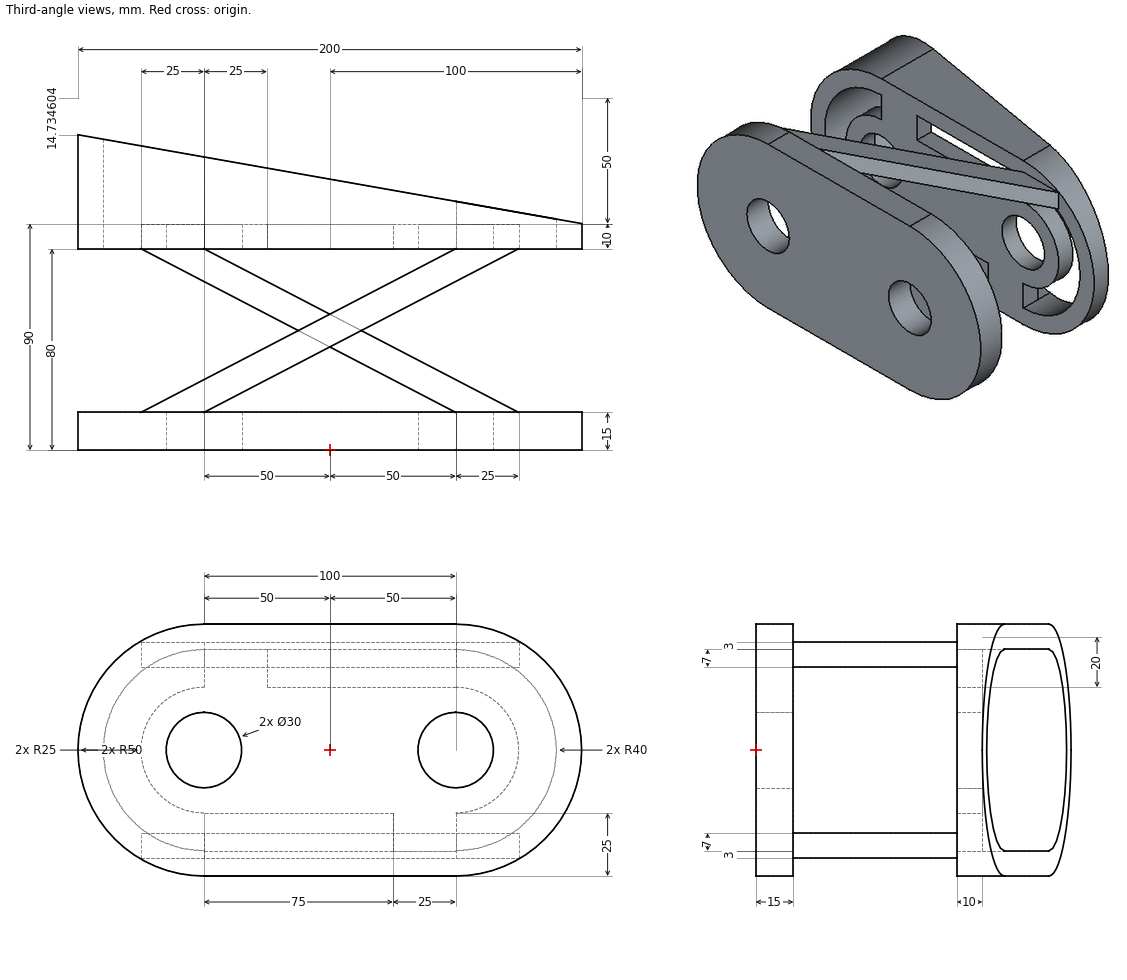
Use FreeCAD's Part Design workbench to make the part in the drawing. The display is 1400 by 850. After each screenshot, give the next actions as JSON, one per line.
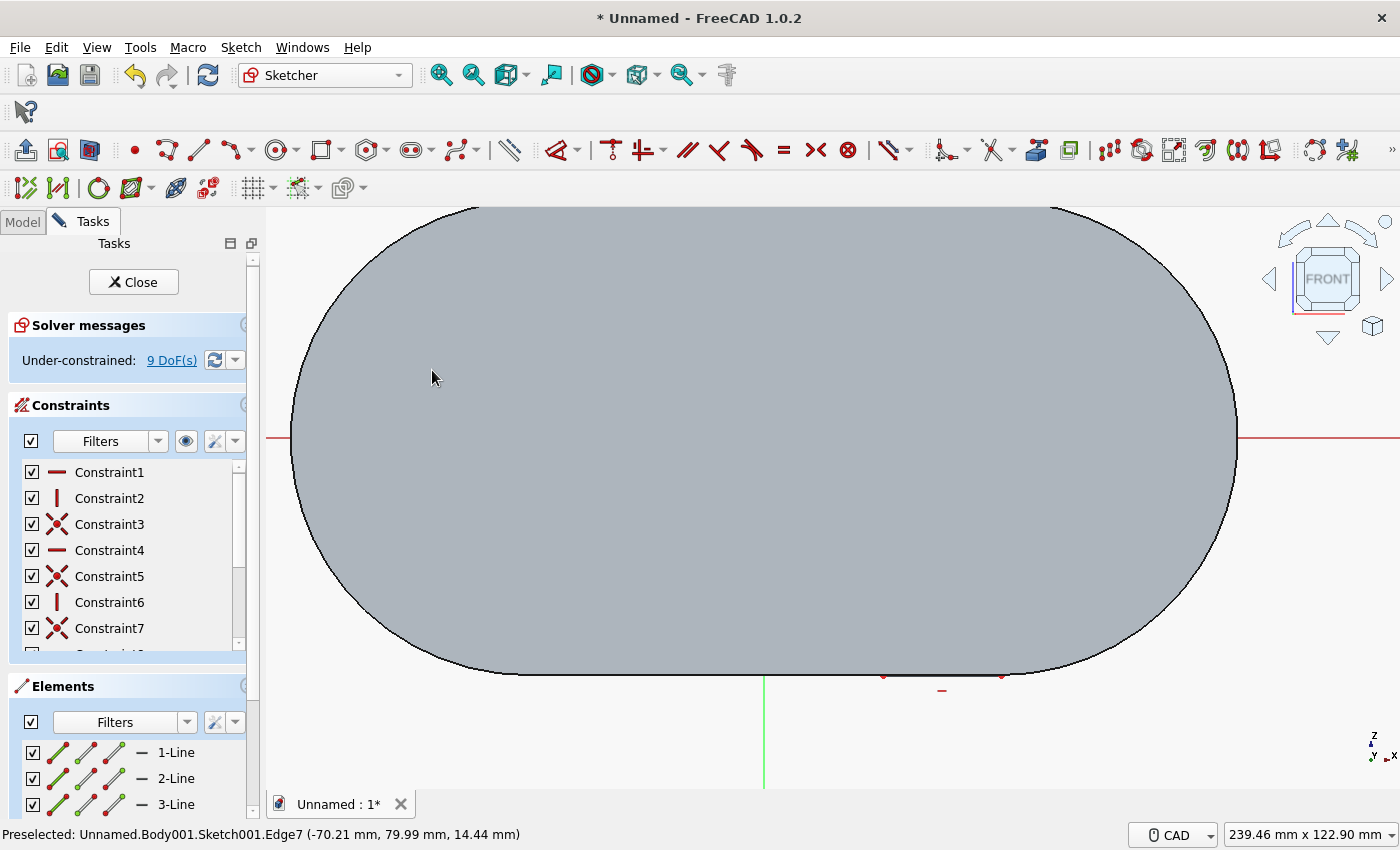
{"action": "left_click", "coordinate": [752, 150]}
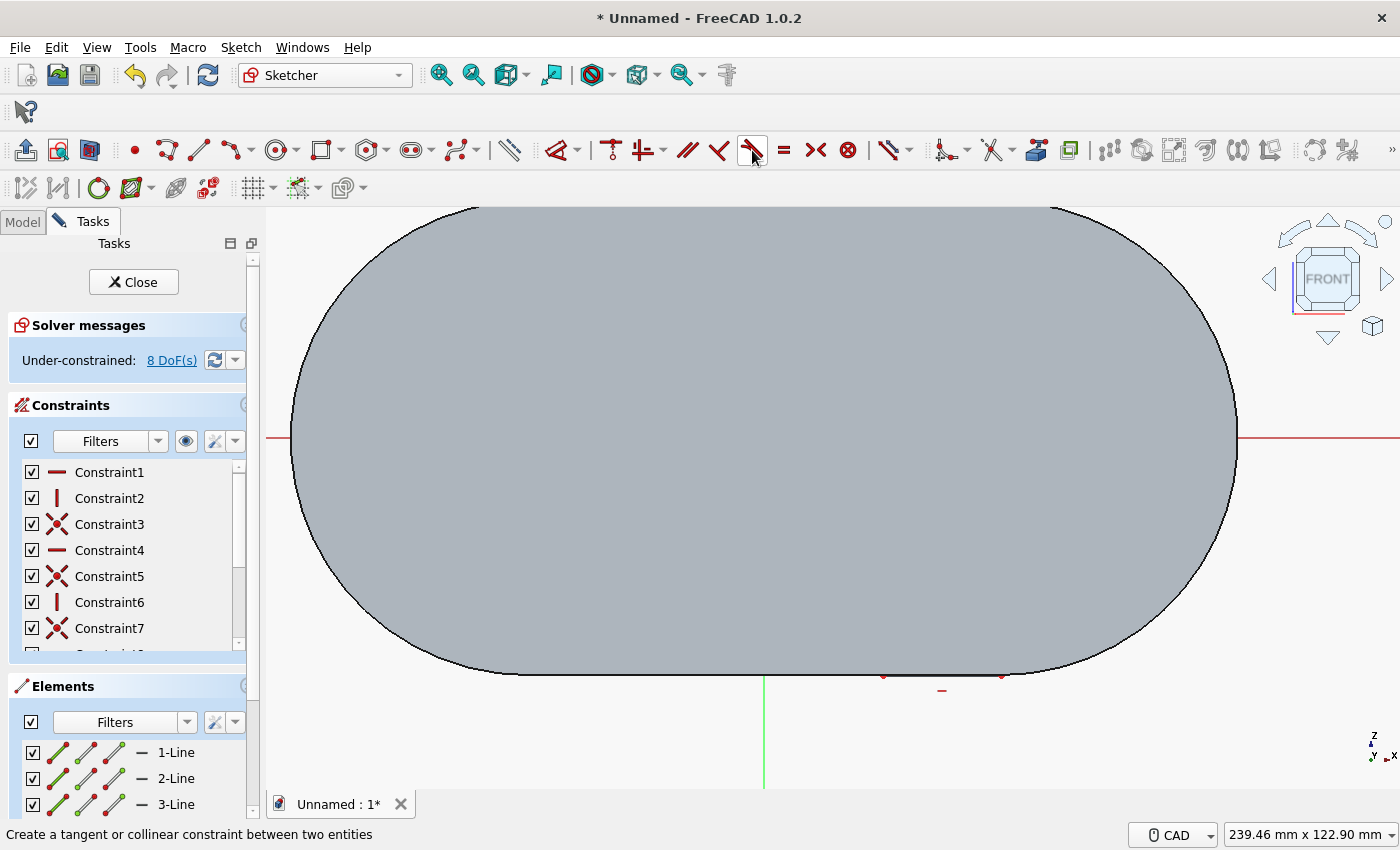
{"action": "left_click", "coordinate": [1097, 509]}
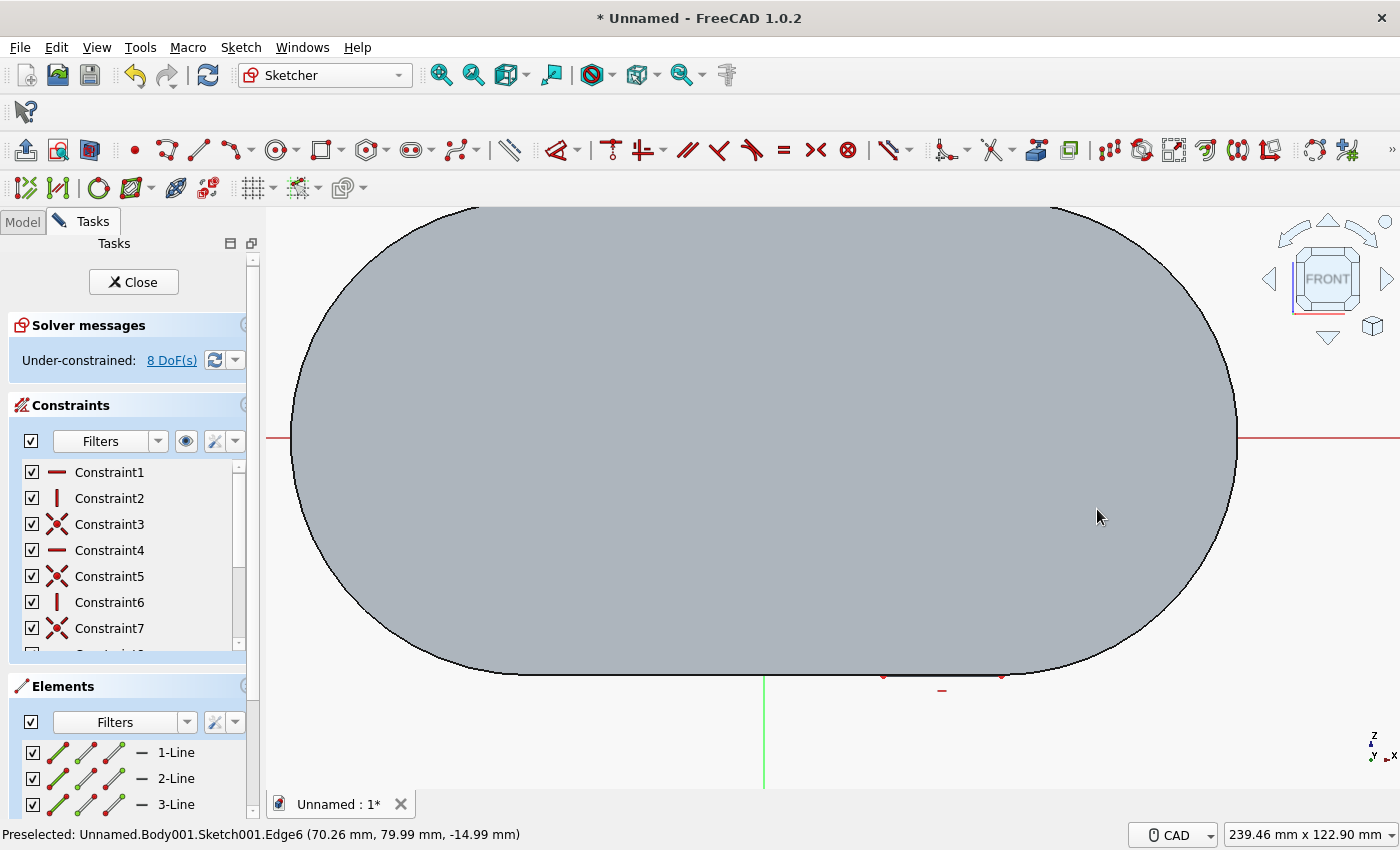
{"action": "left_click", "coordinate": [432, 370]}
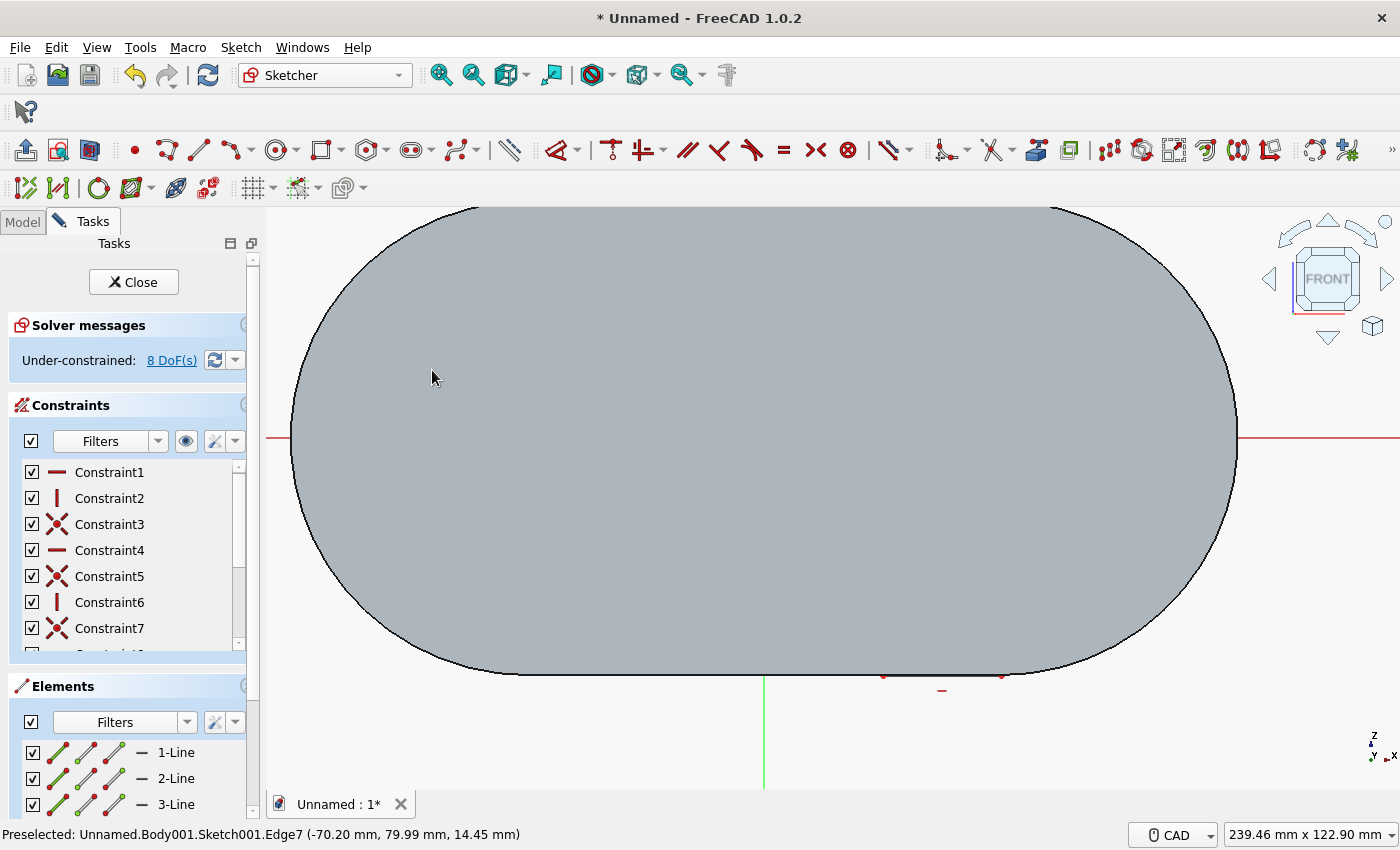
{"action": "left_click", "coordinate": [784, 150]}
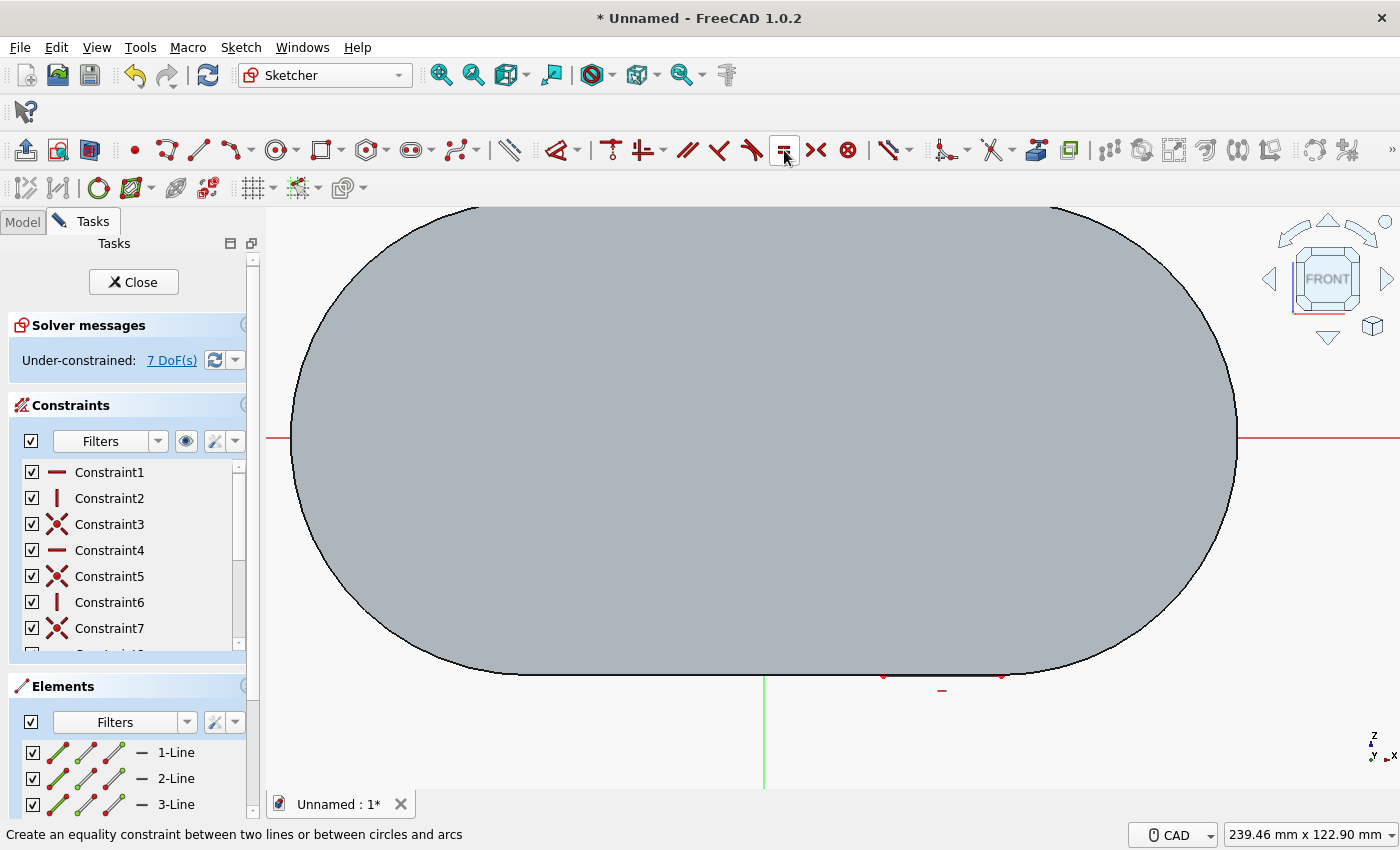
{"action": "left_click", "coordinate": [1001, 440]}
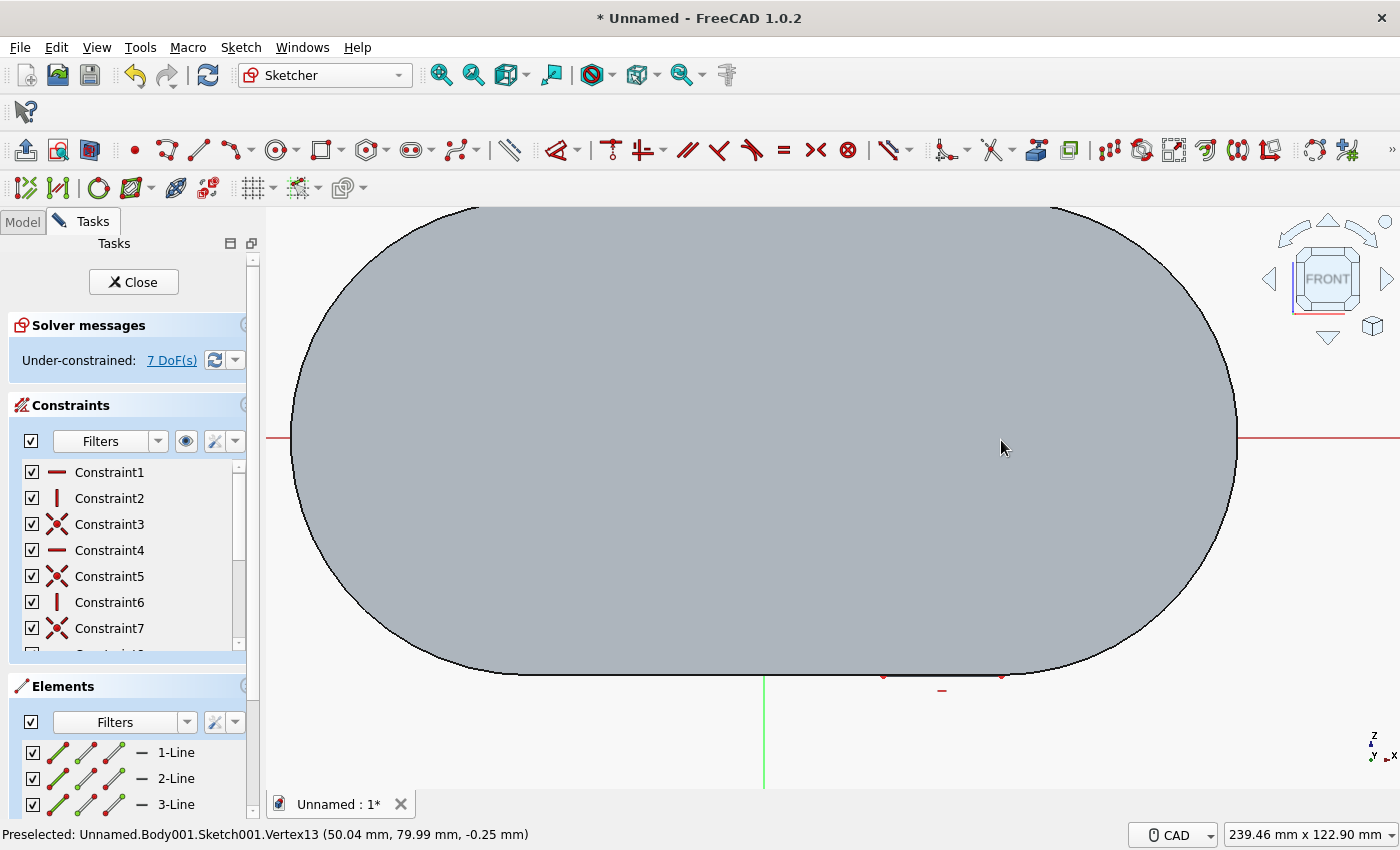
{"action": "left_click", "coordinate": [361, 438]}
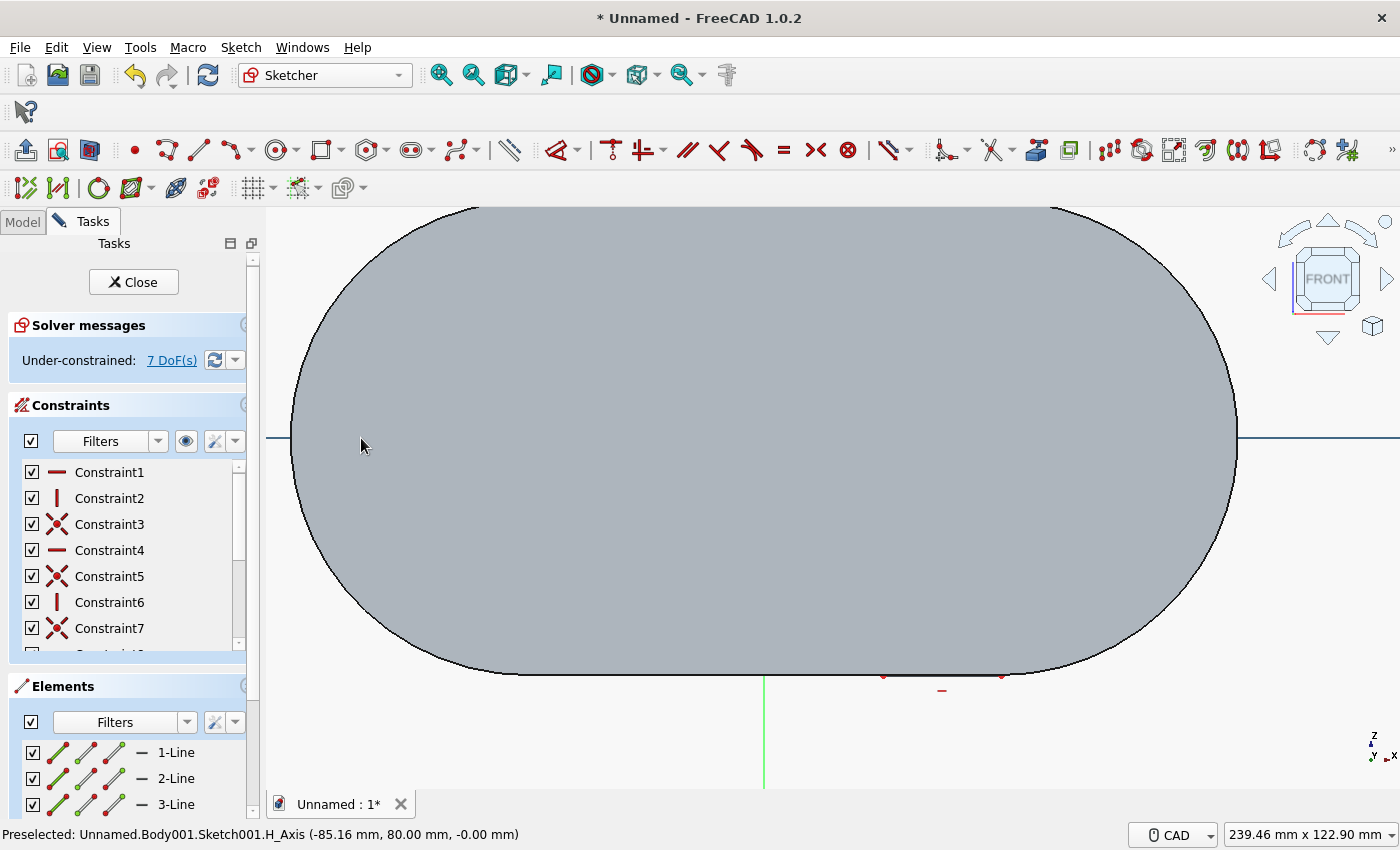
{"action": "left_click", "coordinate": [612, 150]}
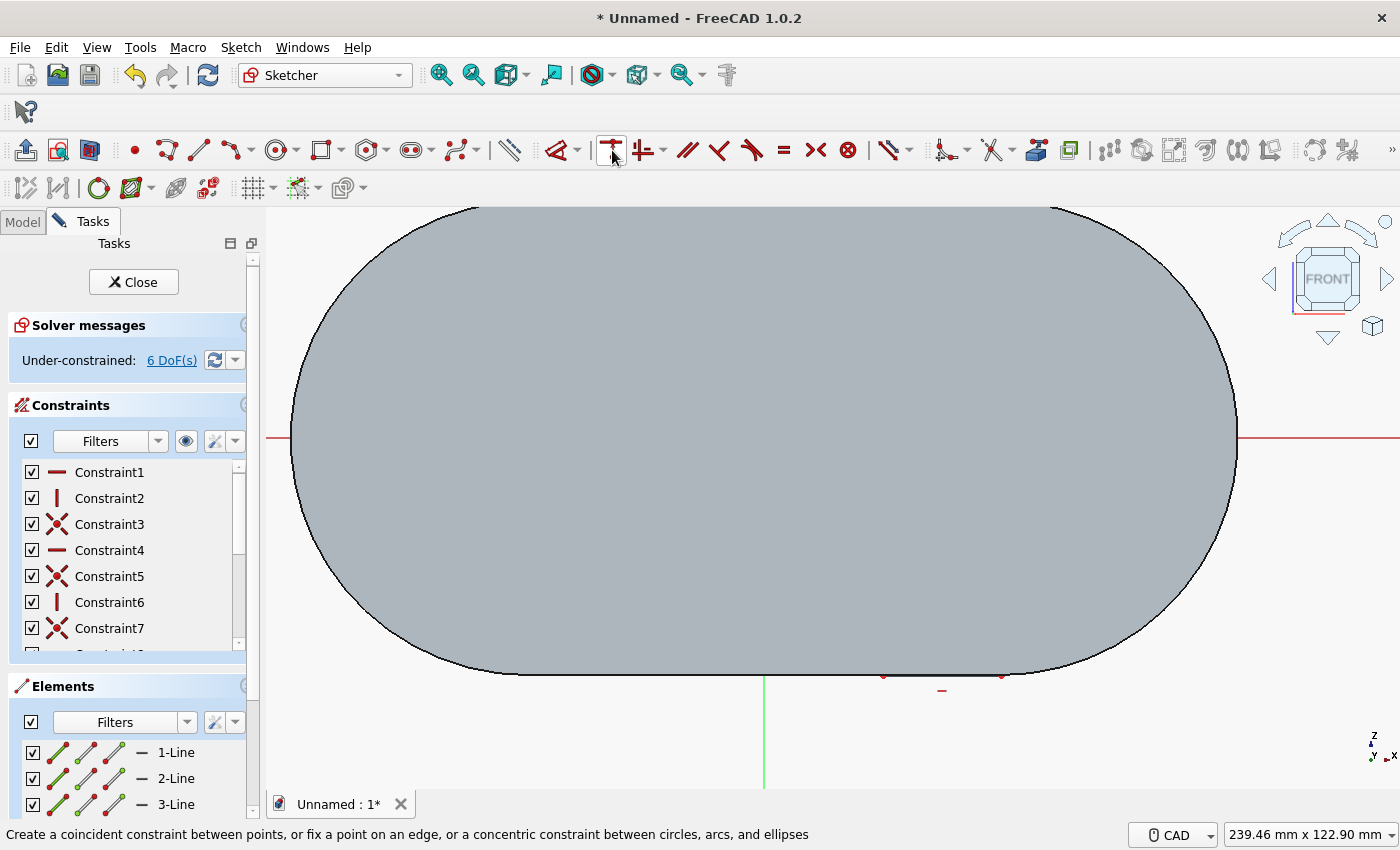
{"action": "left_click", "coordinate": [556, 150]}